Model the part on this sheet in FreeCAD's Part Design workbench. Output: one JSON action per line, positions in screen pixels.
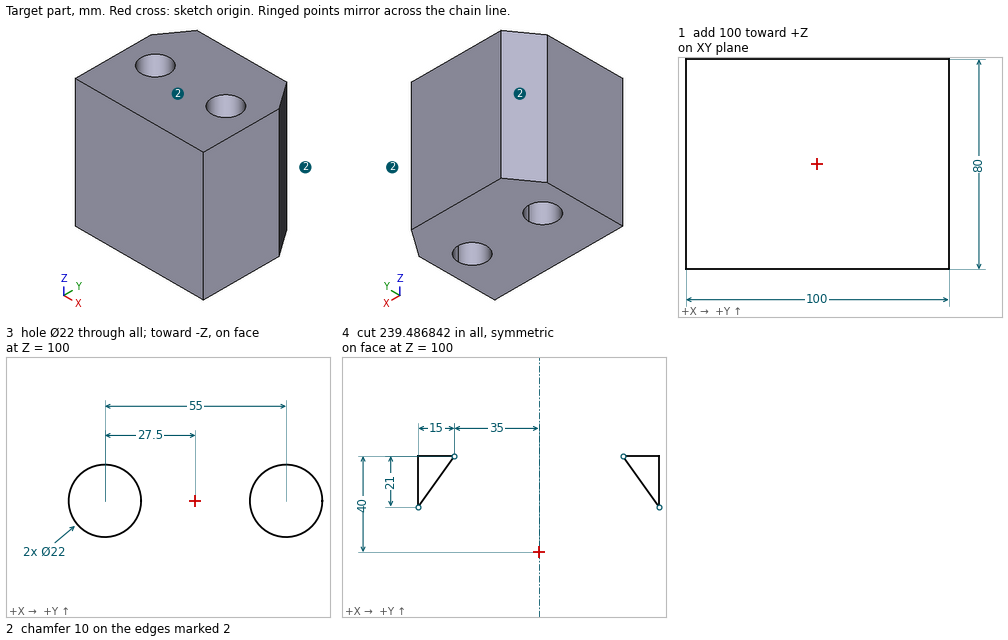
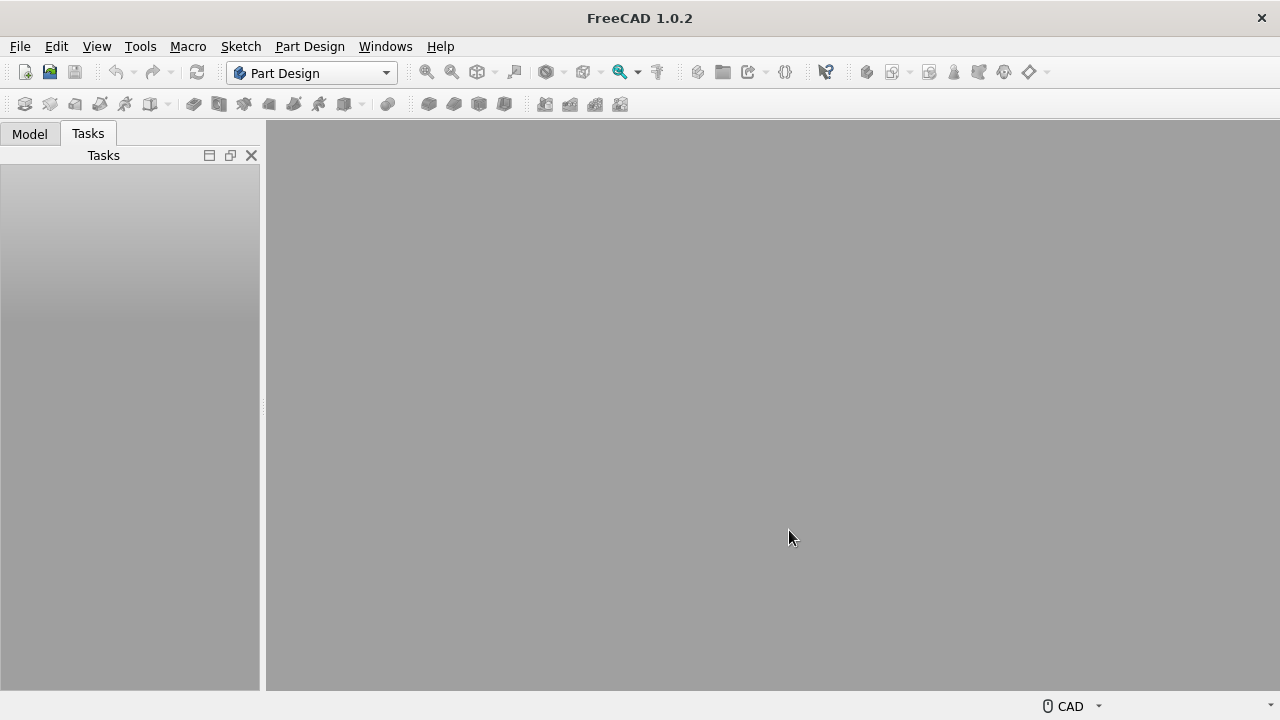
{"action": "left_click", "coordinate": [25, 72]}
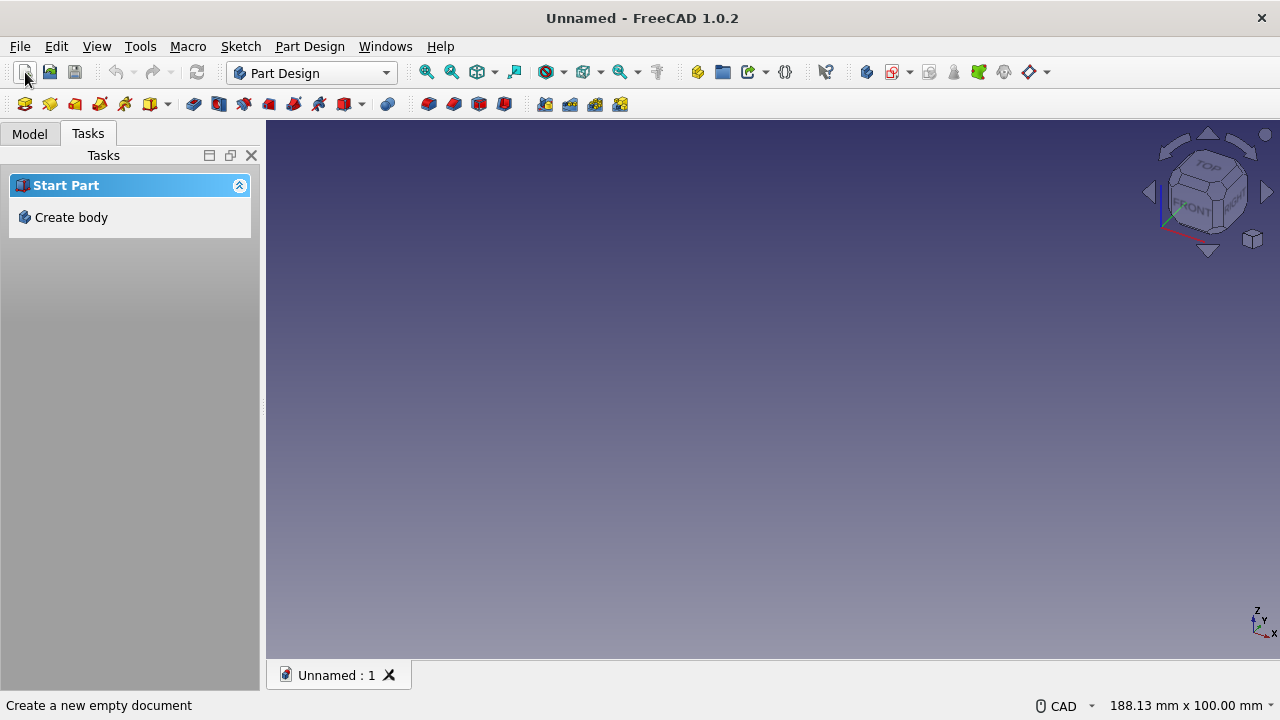
{"action": "left_click", "coordinate": [892, 72]}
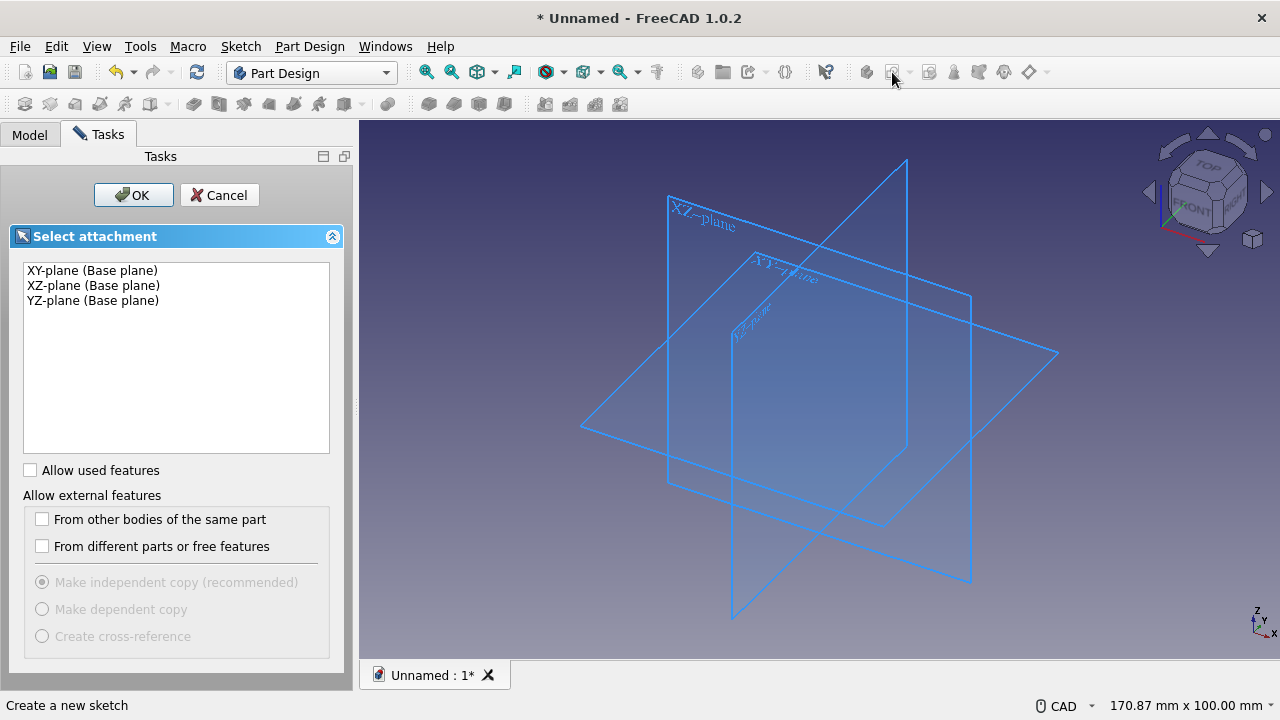
{"action": "left_click", "coordinate": [84, 270]}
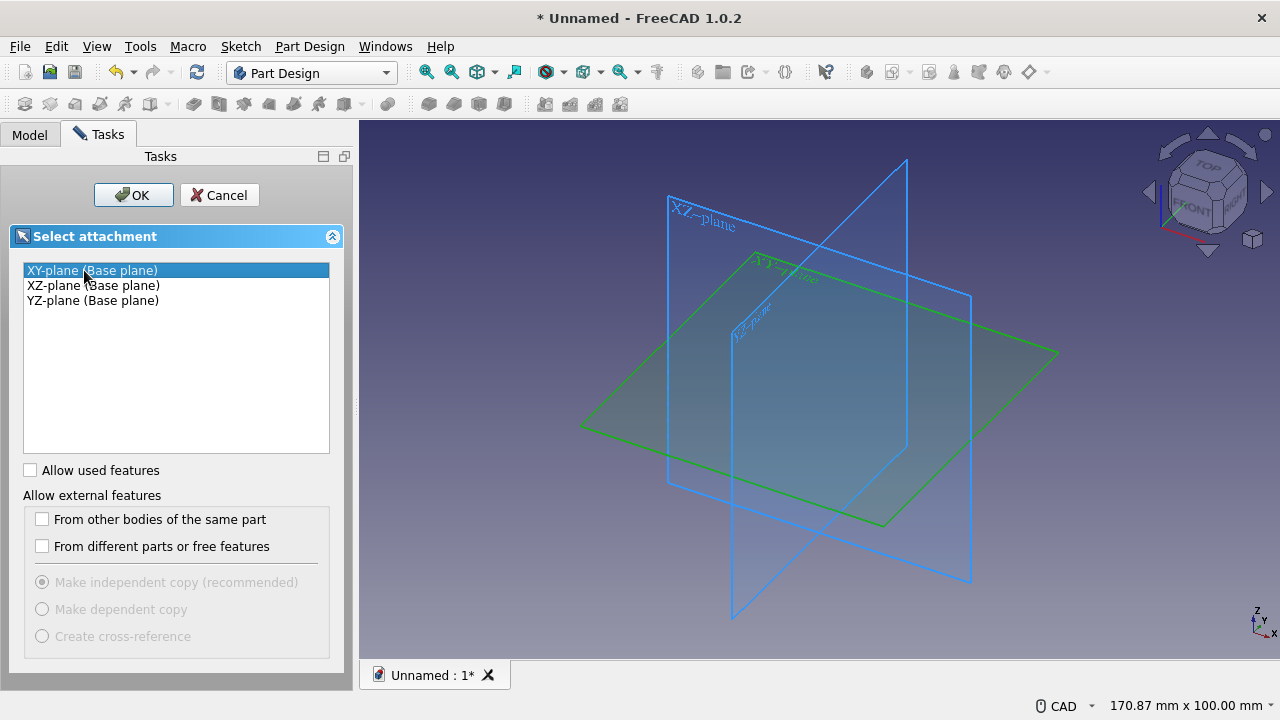
{"action": "left_click", "coordinate": [134, 195]}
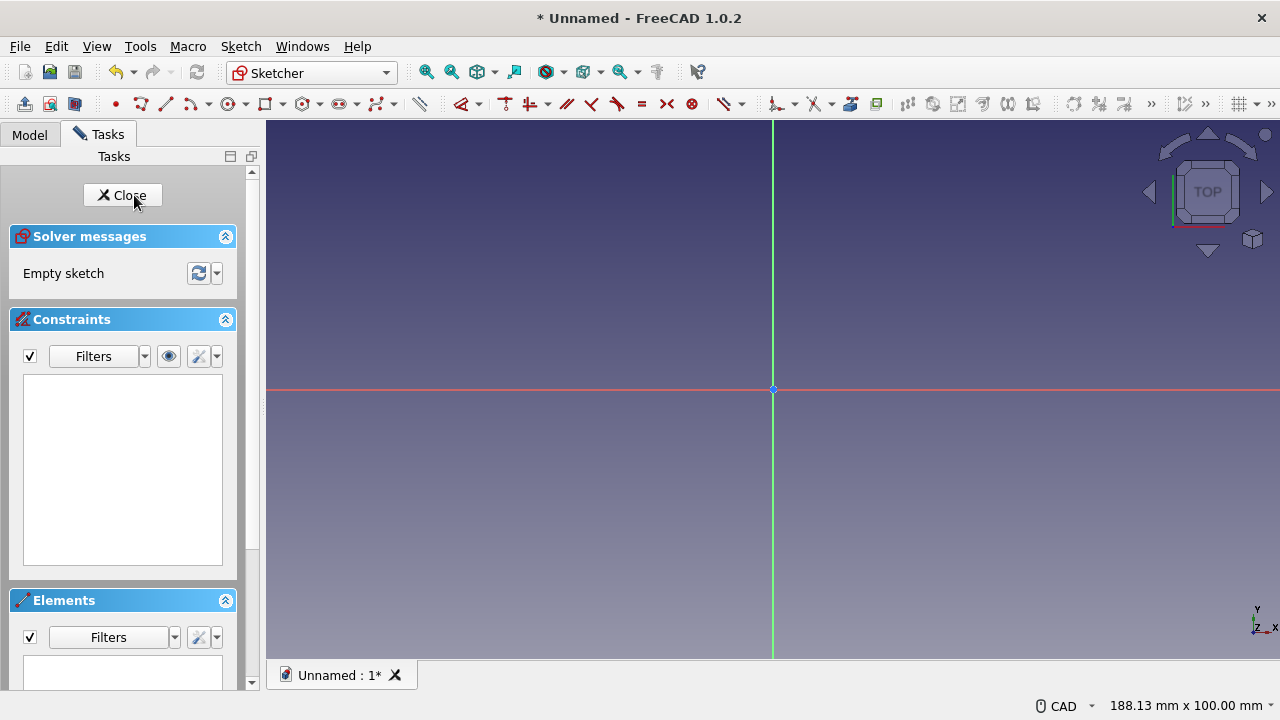
{"action": "left_click", "coordinate": [282, 104]}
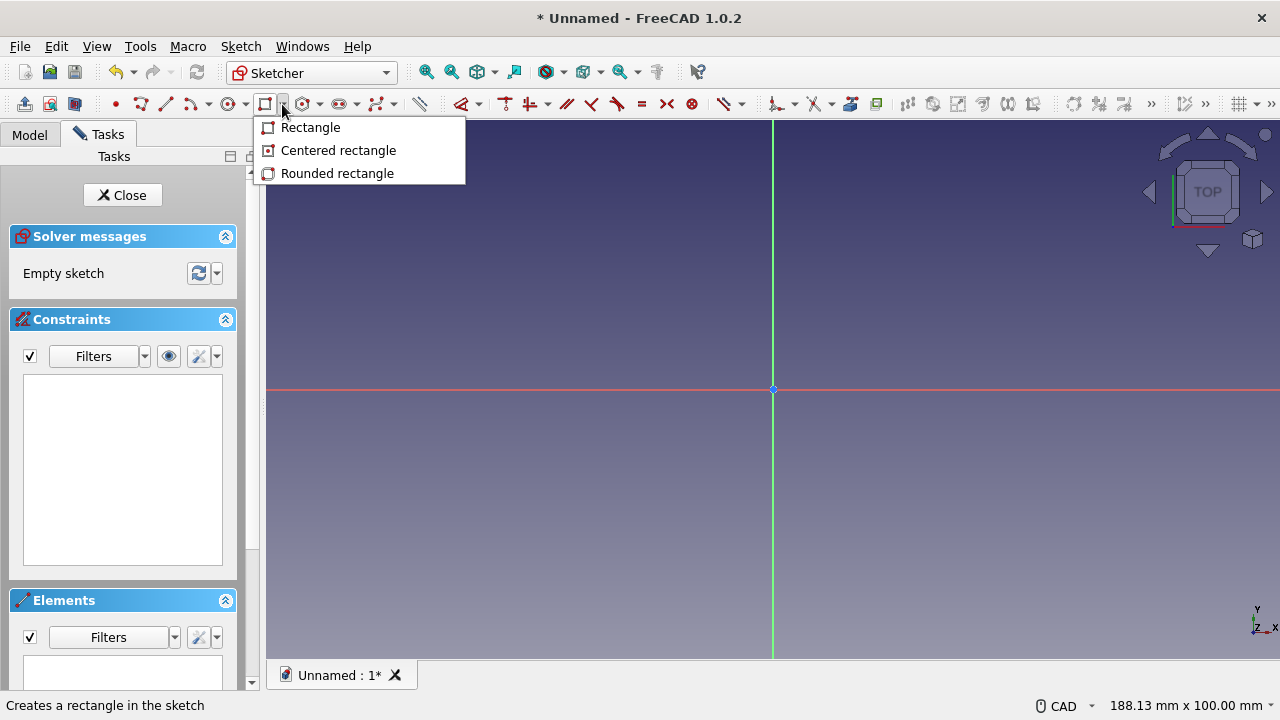
{"action": "left_click", "coordinate": [360, 150]}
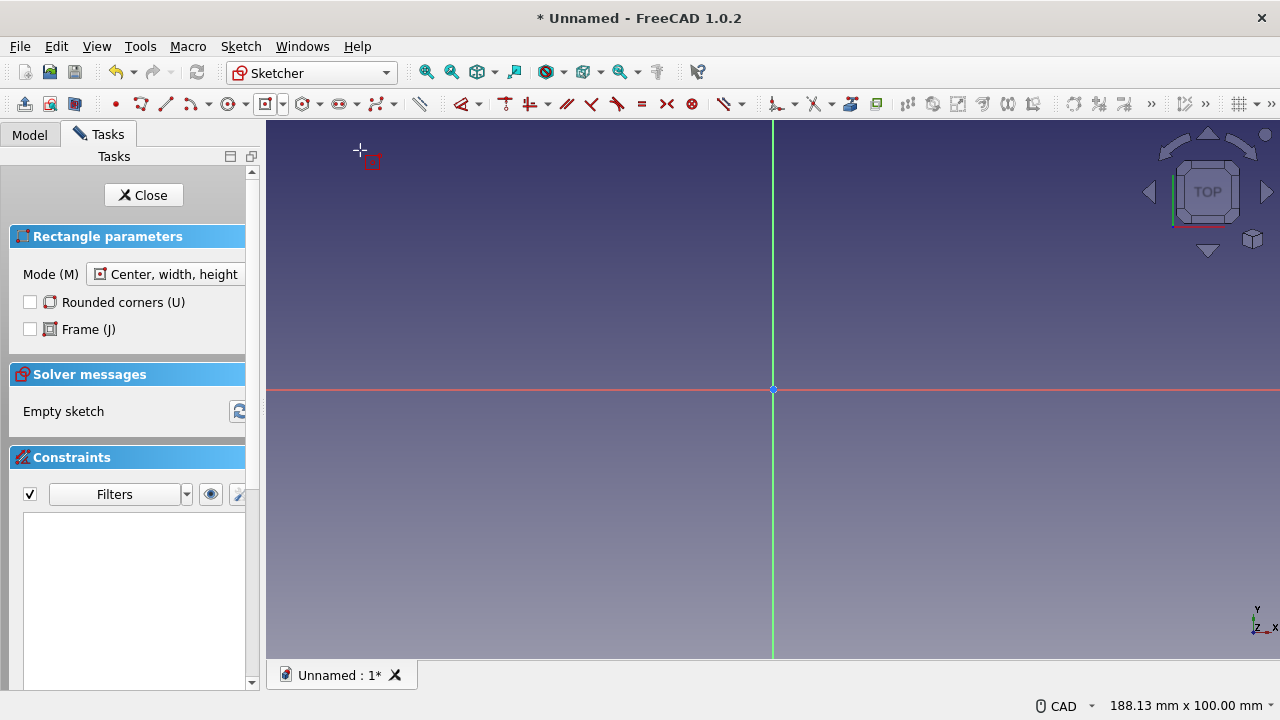
{"action": "left_click", "coordinate": [773, 390]}
{"action": "left_click", "coordinate": [1042, 174]}
{"action": "key", "text": "Escape"}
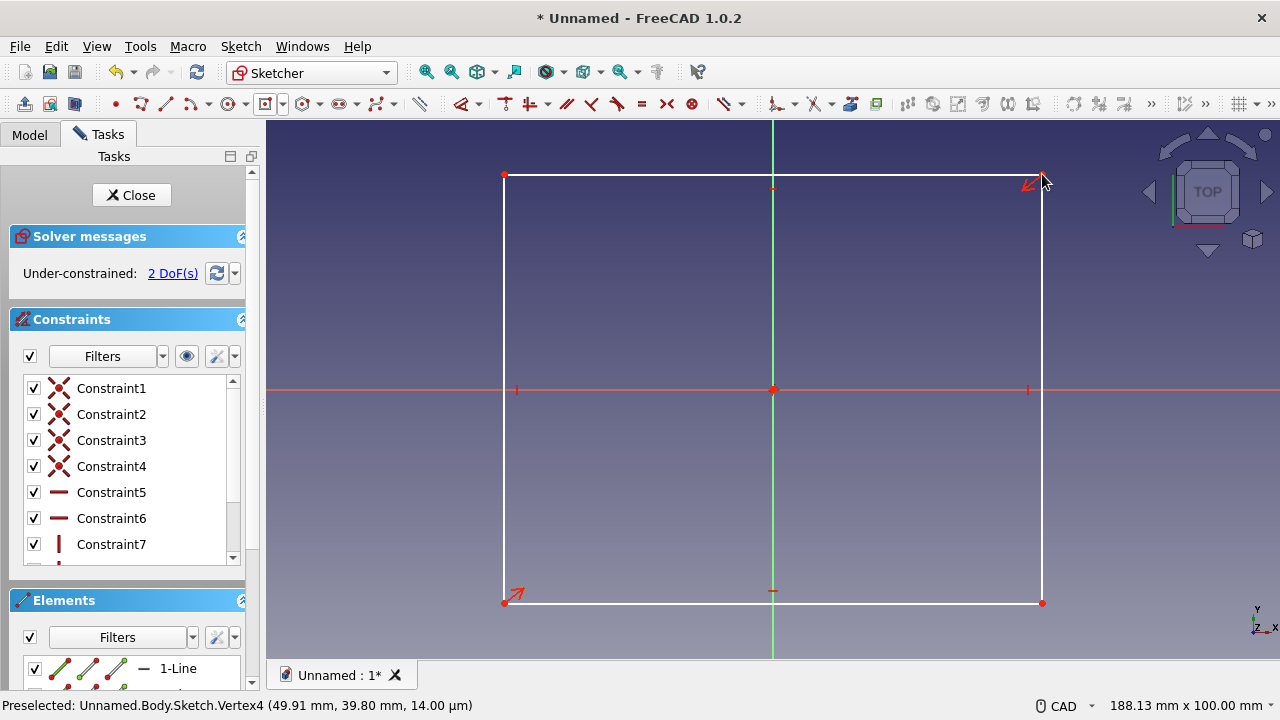
{"action": "left_click", "coordinate": [460, 104]}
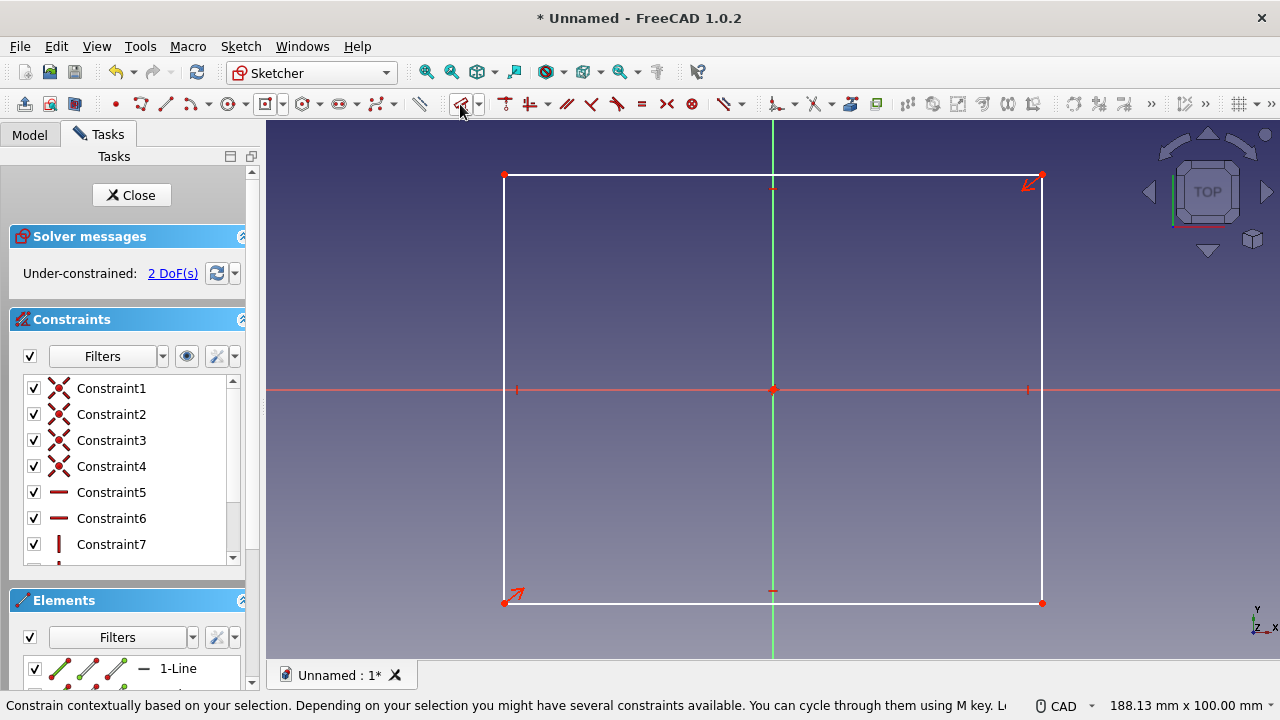
{"action": "left_click", "coordinate": [1042, 475]}
{"action": "left_click", "coordinate": [1076, 291]}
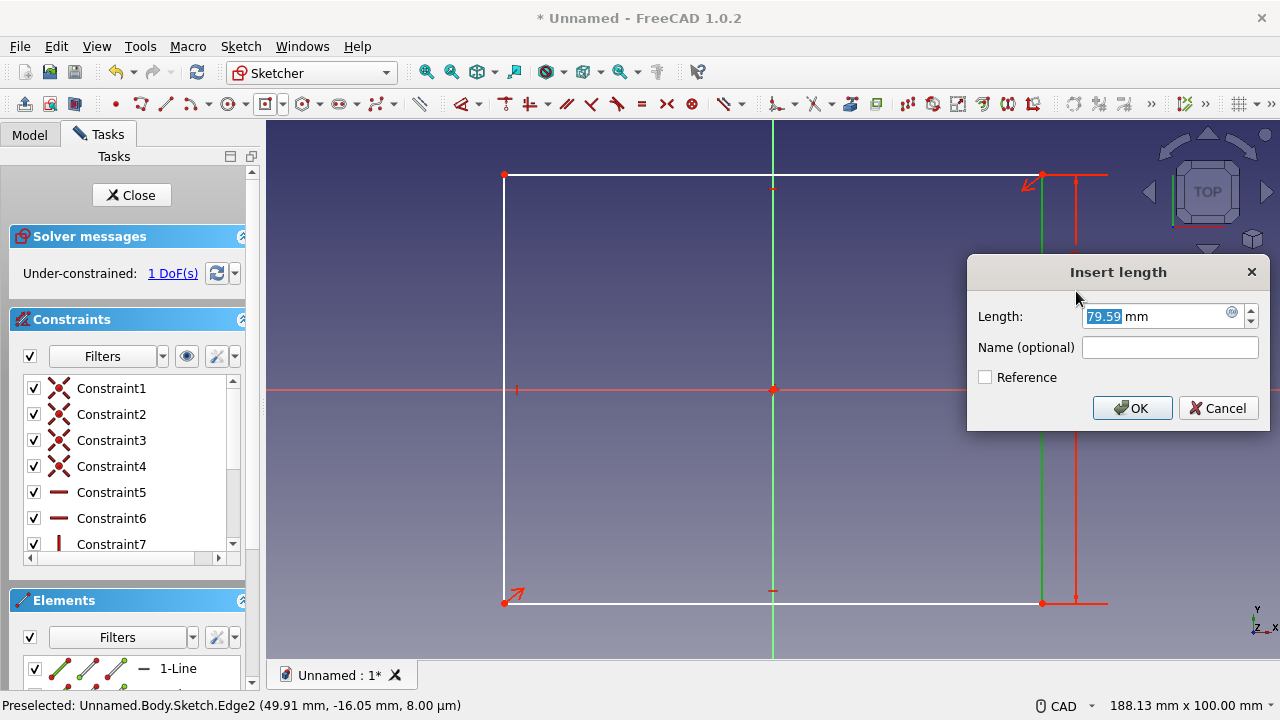
{"action": "type", "text": "80"}
{"action": "key", "text": "Return"}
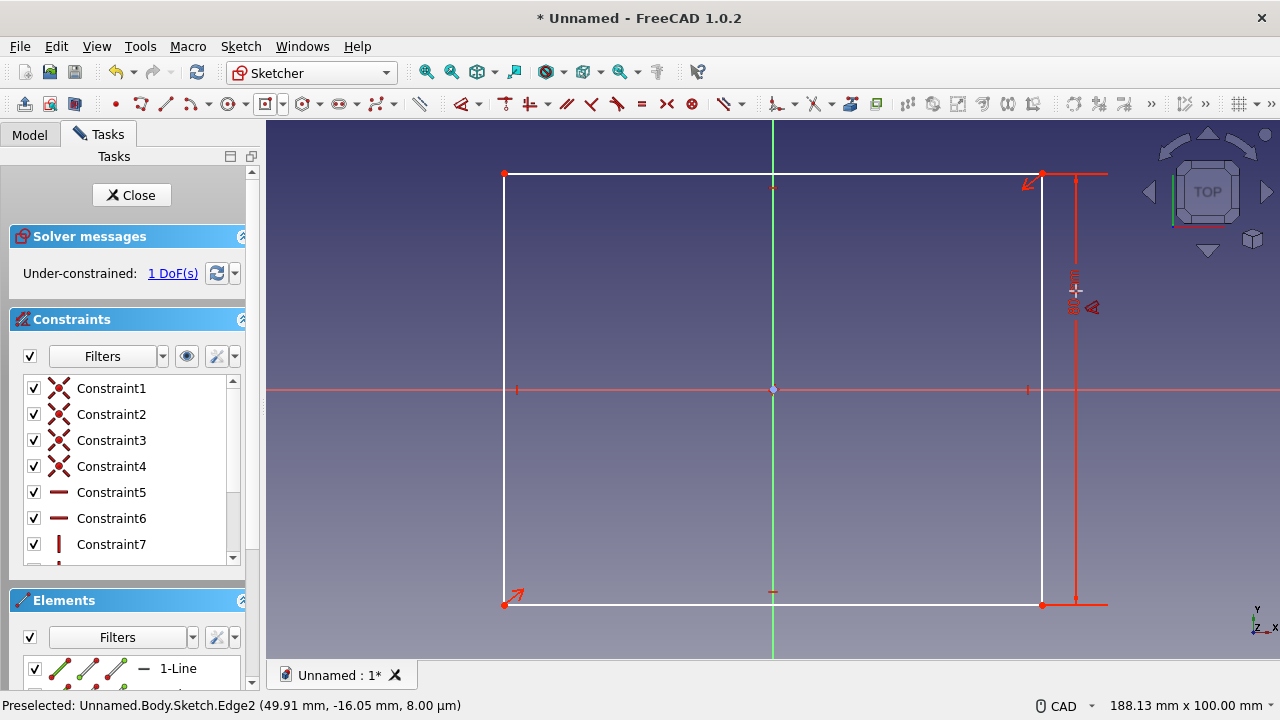
{"action": "left_click", "coordinate": [665, 605]}
{"action": "left_click", "coordinate": [649, 571]}